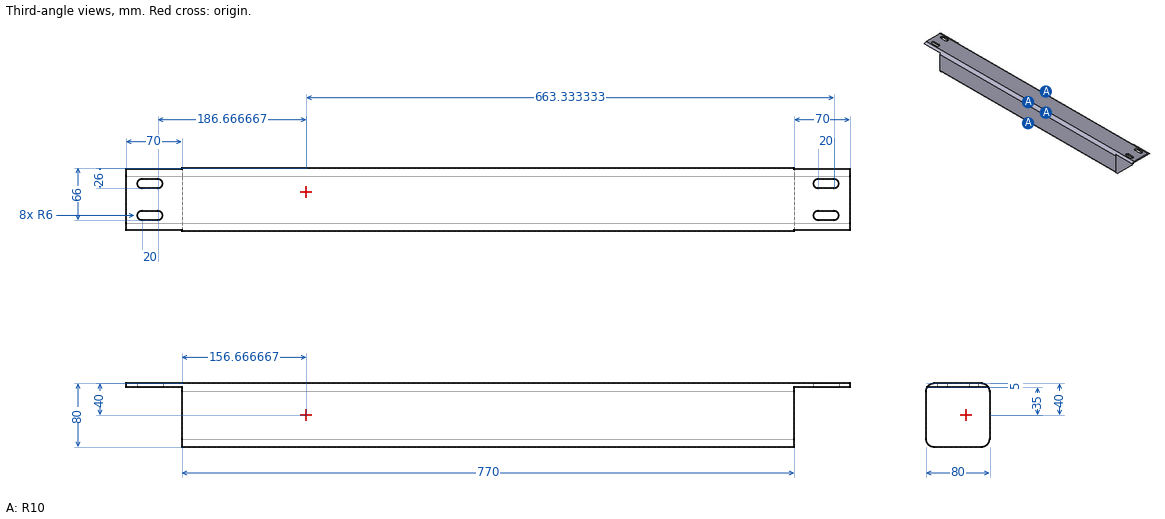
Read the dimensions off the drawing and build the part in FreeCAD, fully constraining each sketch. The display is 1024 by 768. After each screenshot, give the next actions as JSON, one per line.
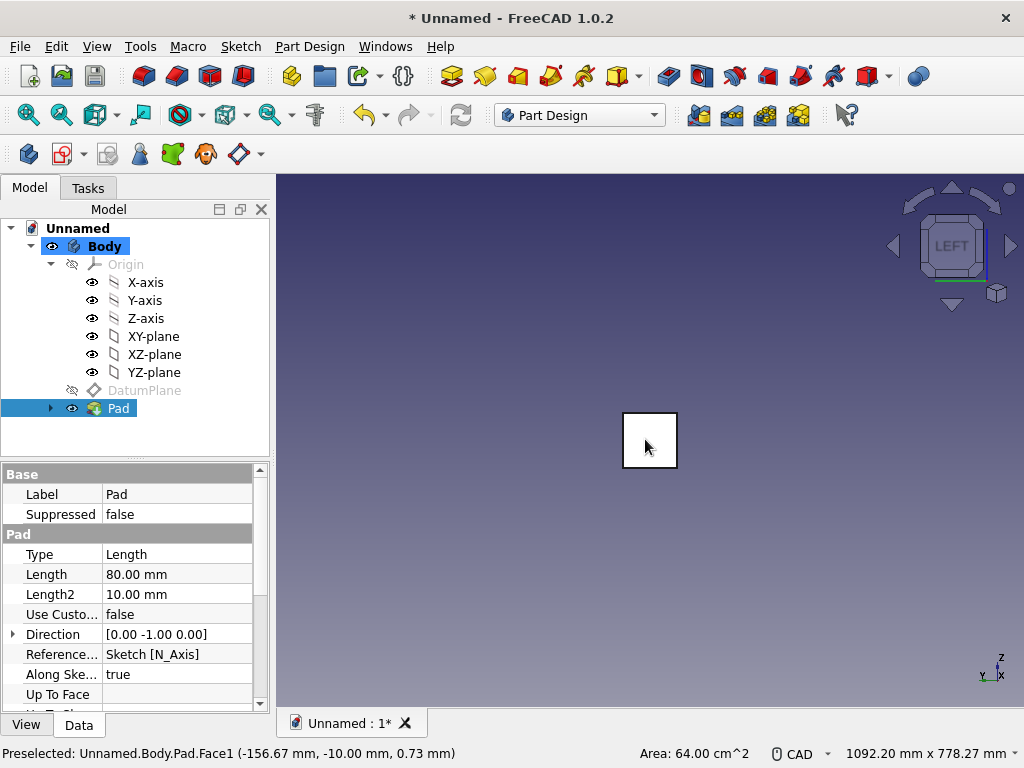
{"action": "left_click", "coordinate": [62, 154]}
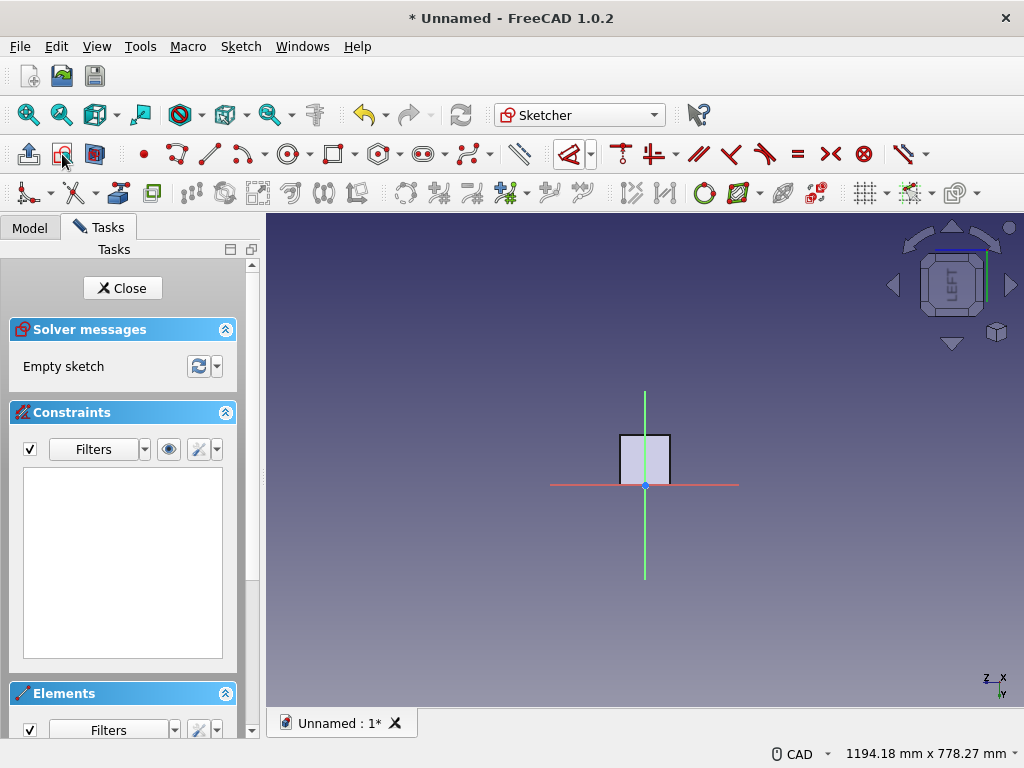
{"action": "scroll", "coordinate": [643, 460], "scroll_direction": "up", "scroll_amount": 9}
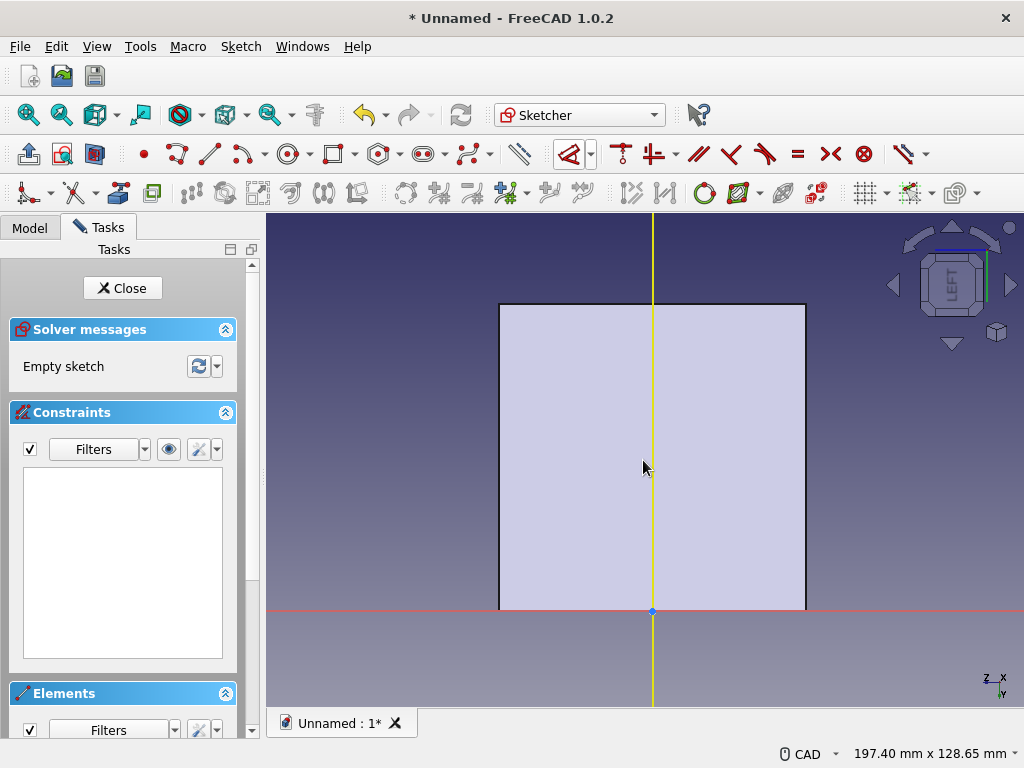
{"action": "left_click", "coordinate": [332, 154]}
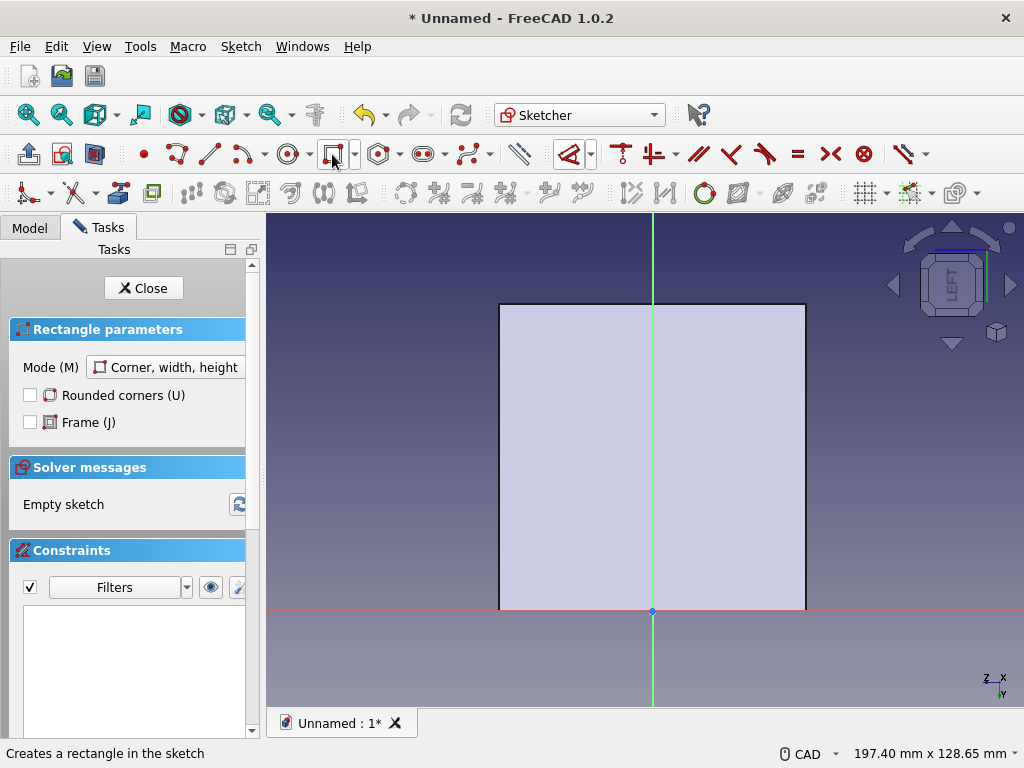
{"action": "left_click", "coordinate": [499, 304]}
{"action": "left_click", "coordinate": [518, 611]}
{"action": "key", "text": "Escape"}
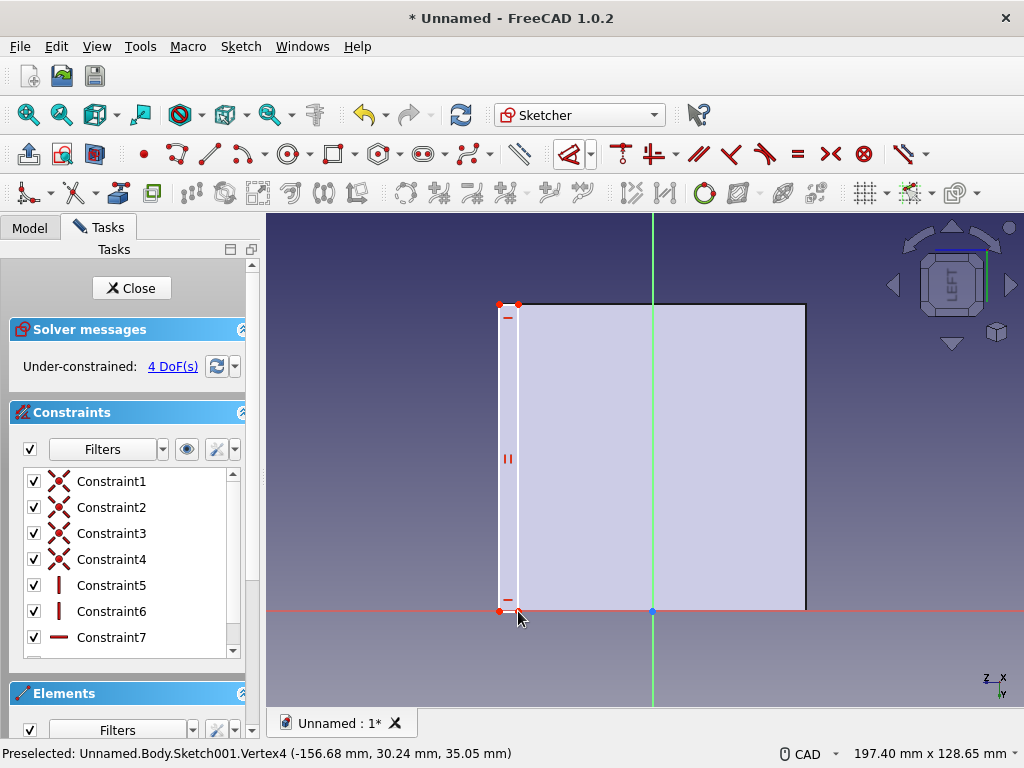
{"action": "left_click", "coordinate": [499, 612]}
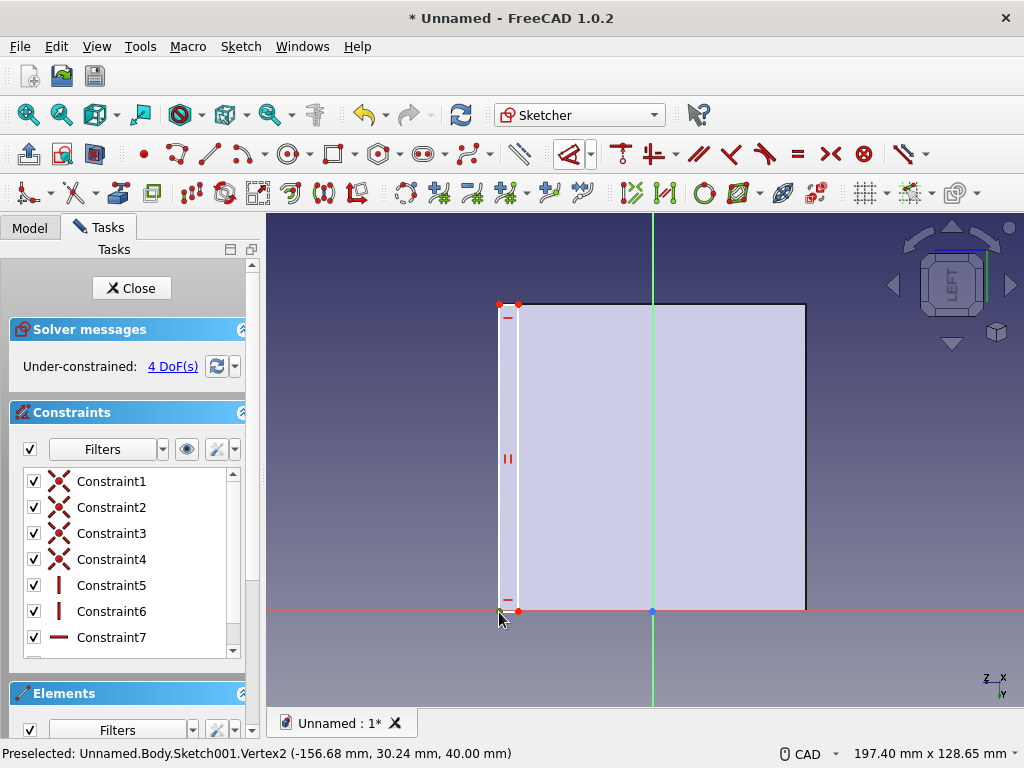
{"action": "left_click", "coordinate": [334, 611]}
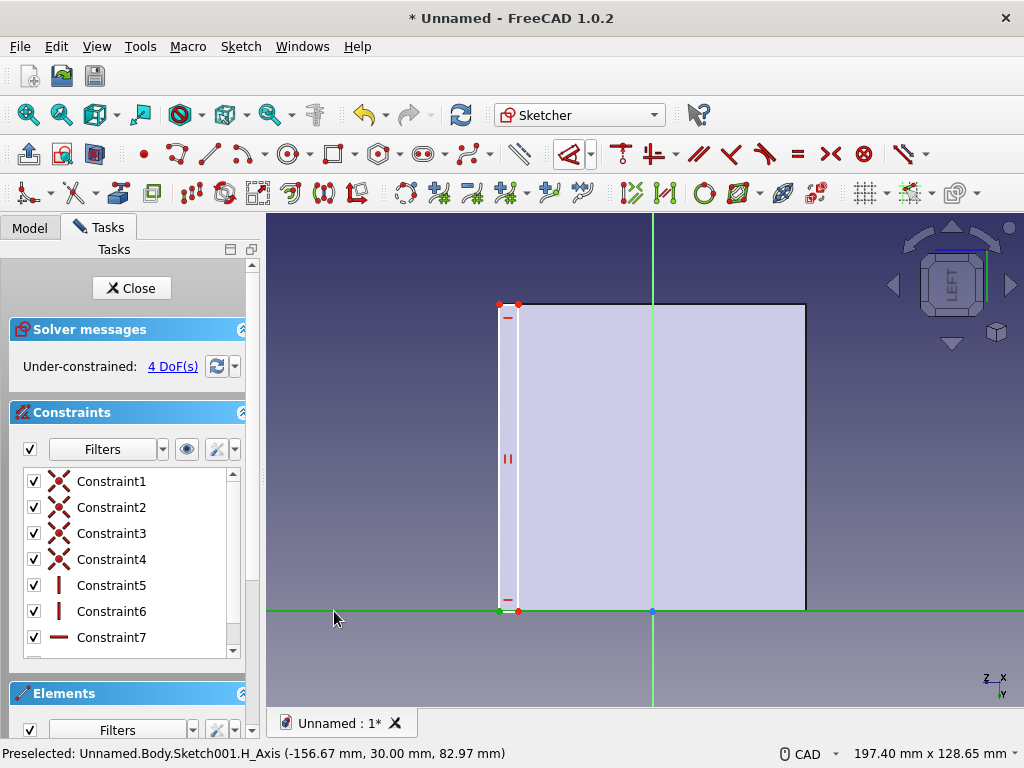
{"action": "left_click", "coordinate": [621, 154]}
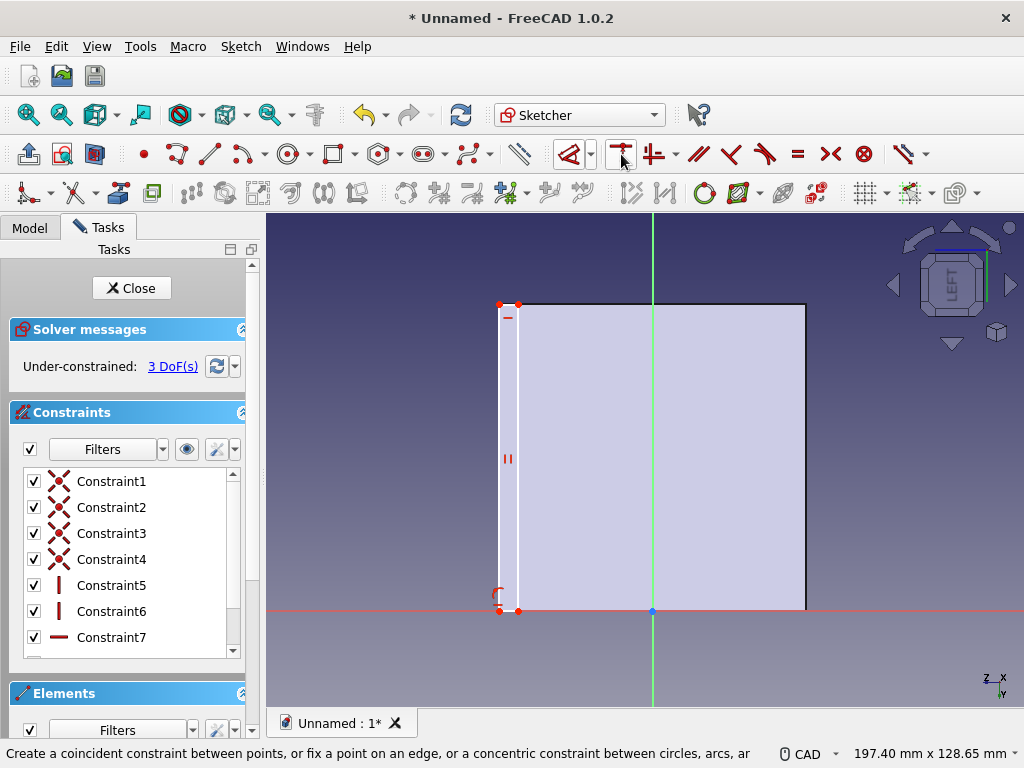
{"action": "scroll", "coordinate": [508, 611], "scroll_direction": "up", "scroll_amount": 4}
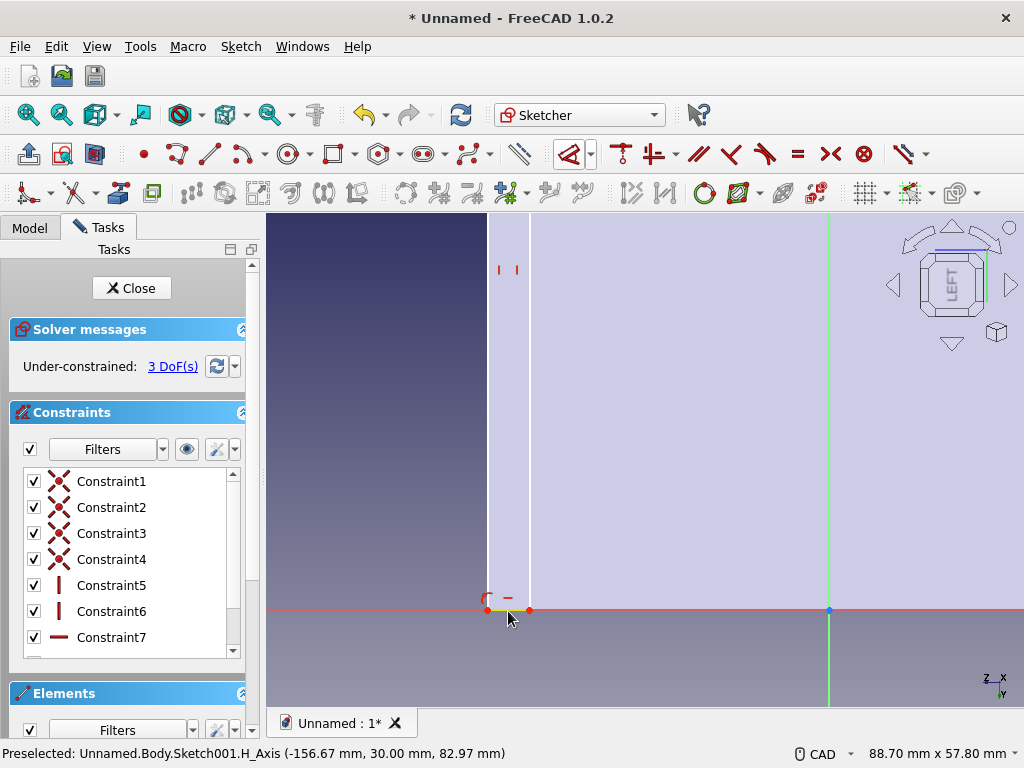
{"action": "left_click", "coordinate": [509, 610]}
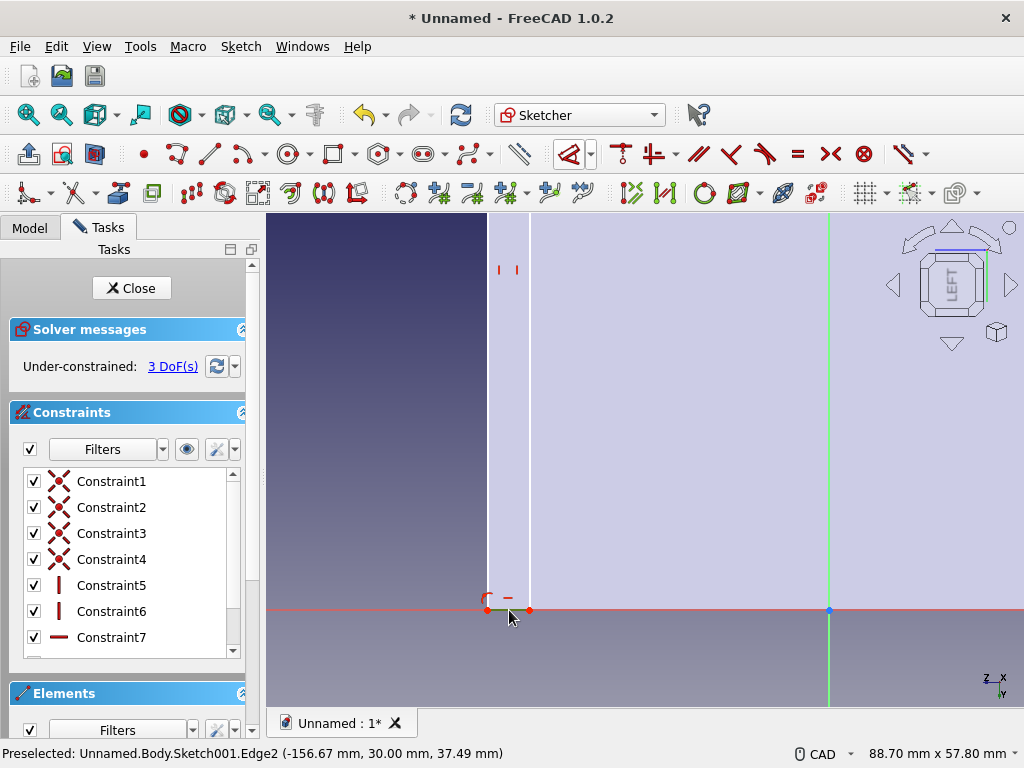
{"action": "key", "text": "l"}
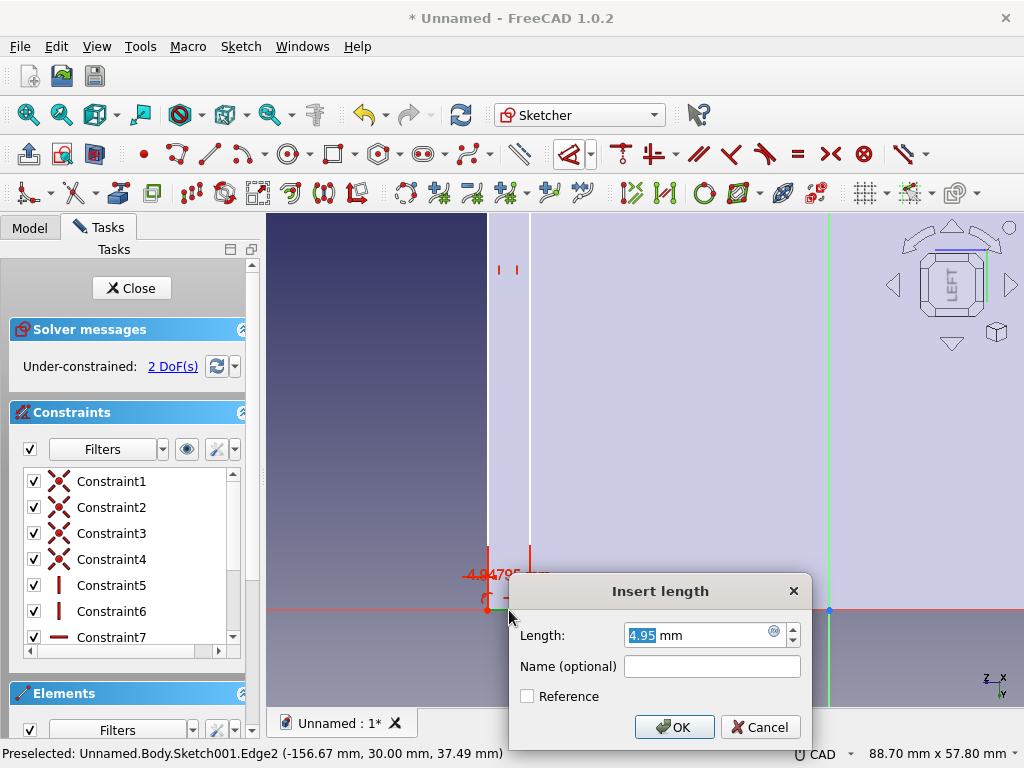
{"action": "type", "text": "5"}
{"action": "key", "text": "Return"}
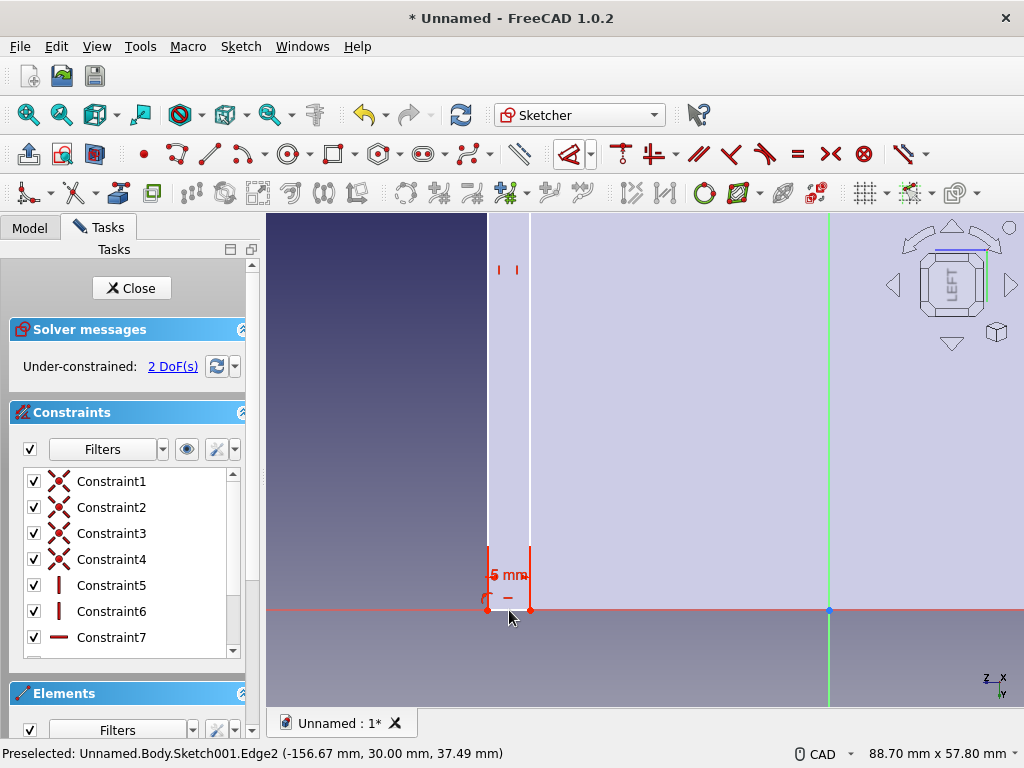
{"action": "left_click", "coordinate": [488, 406]}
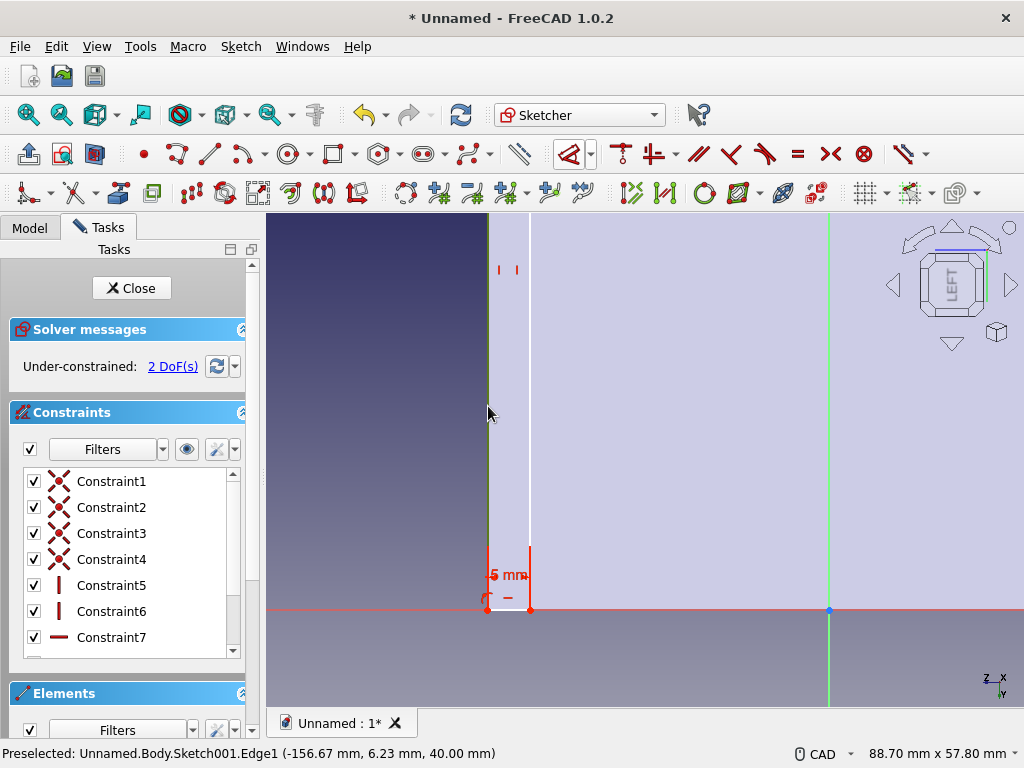
{"action": "left_click", "coordinate": [590, 154]}